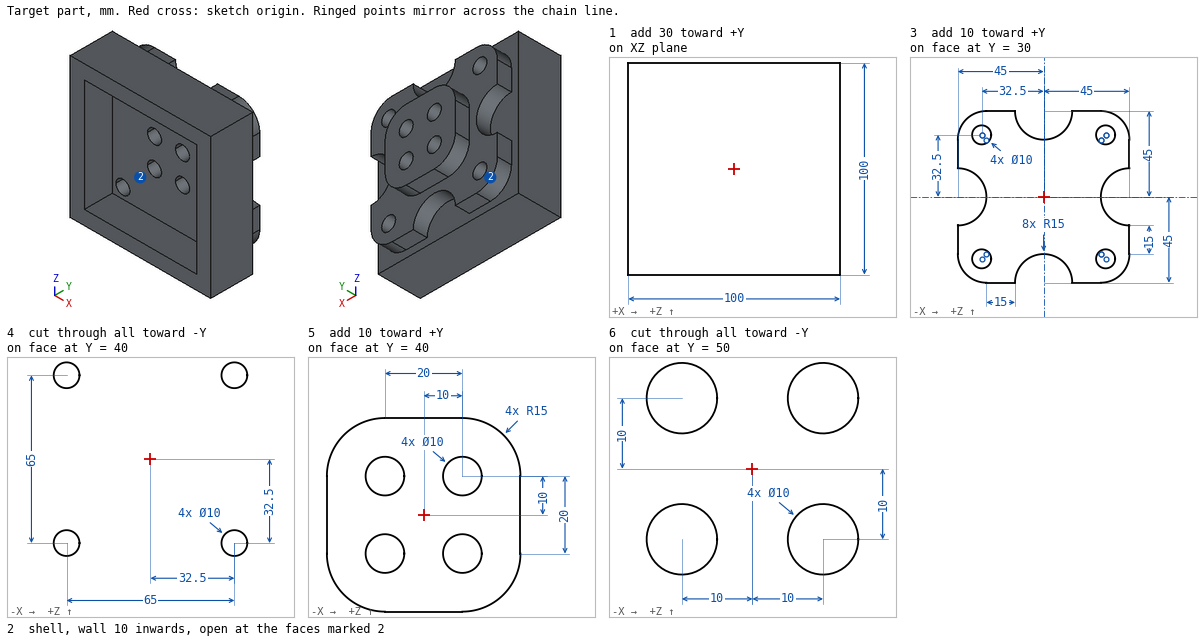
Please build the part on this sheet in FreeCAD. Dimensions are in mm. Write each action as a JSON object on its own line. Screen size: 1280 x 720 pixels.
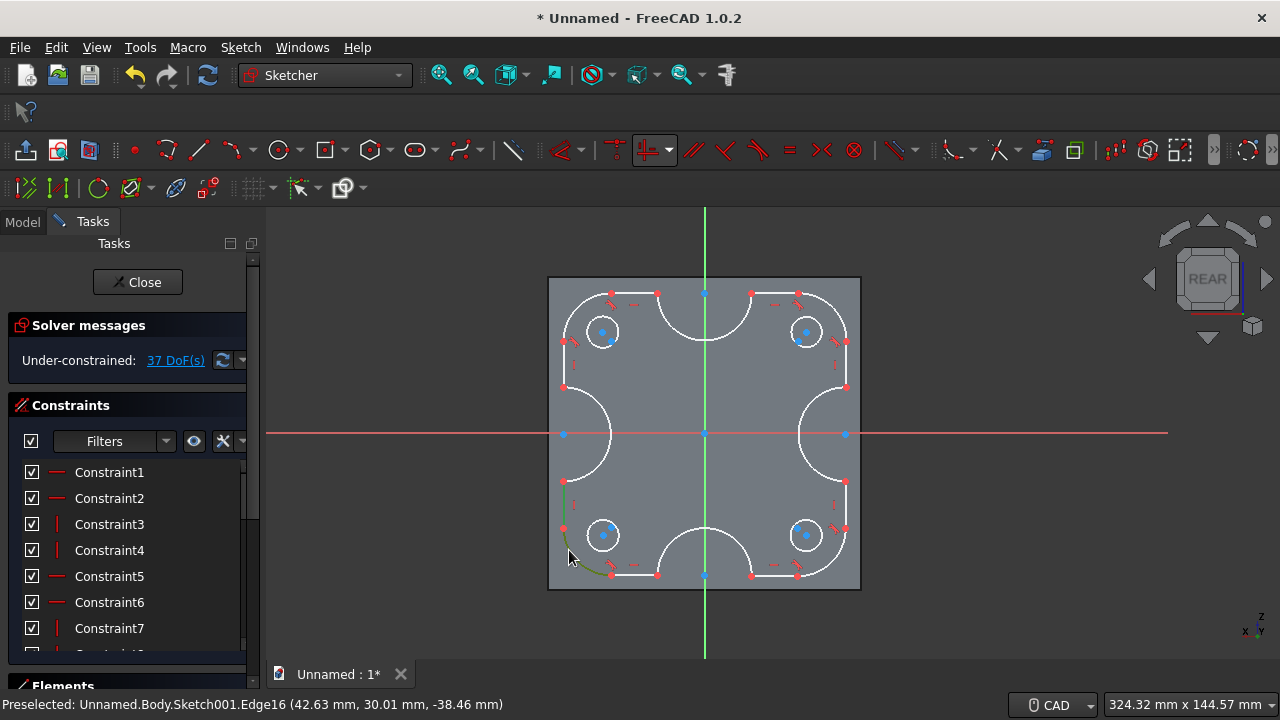
{"action": "left_click", "coordinate": [758, 150]}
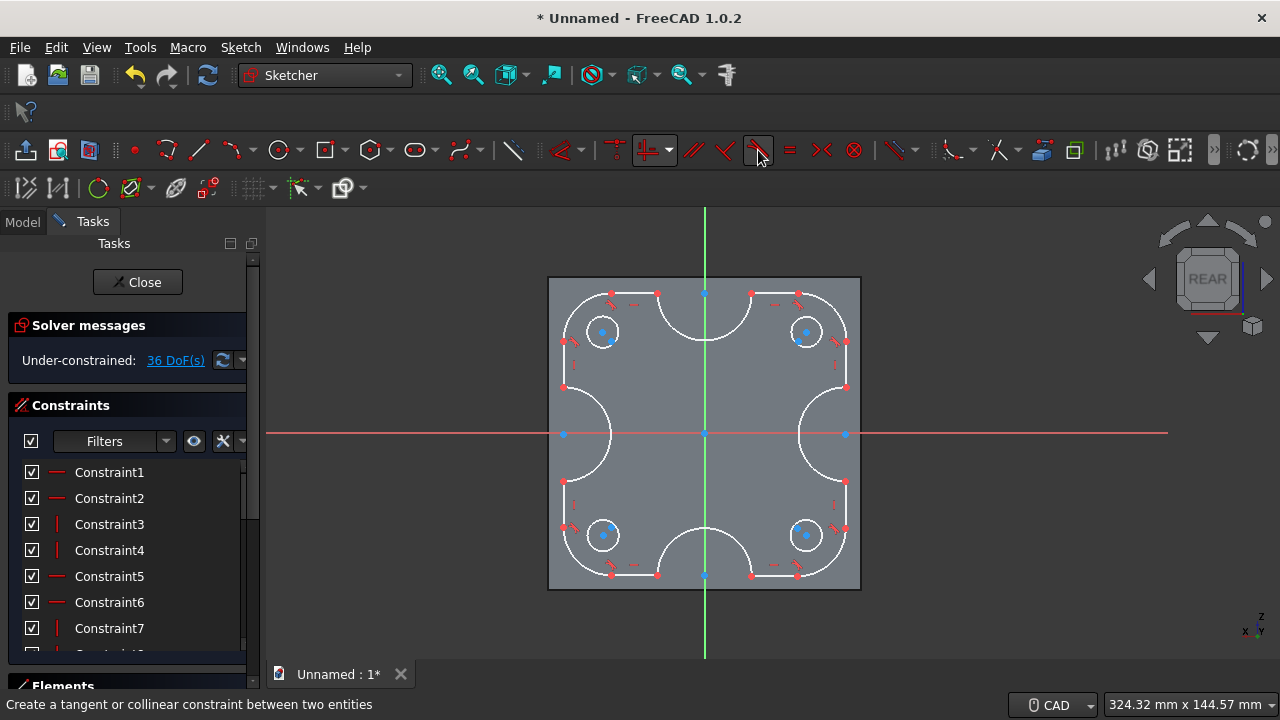
{"action": "left_click", "coordinate": [733, 538]}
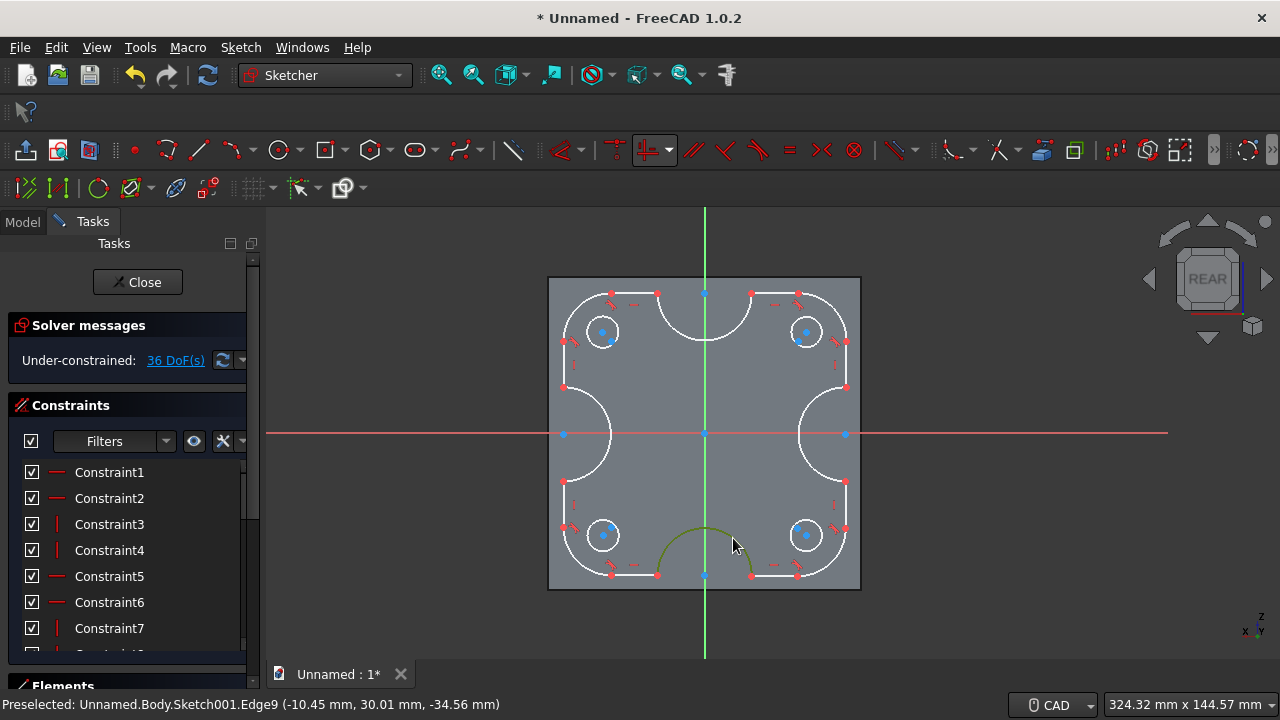
{"action": "left_click", "coordinate": [820, 571]}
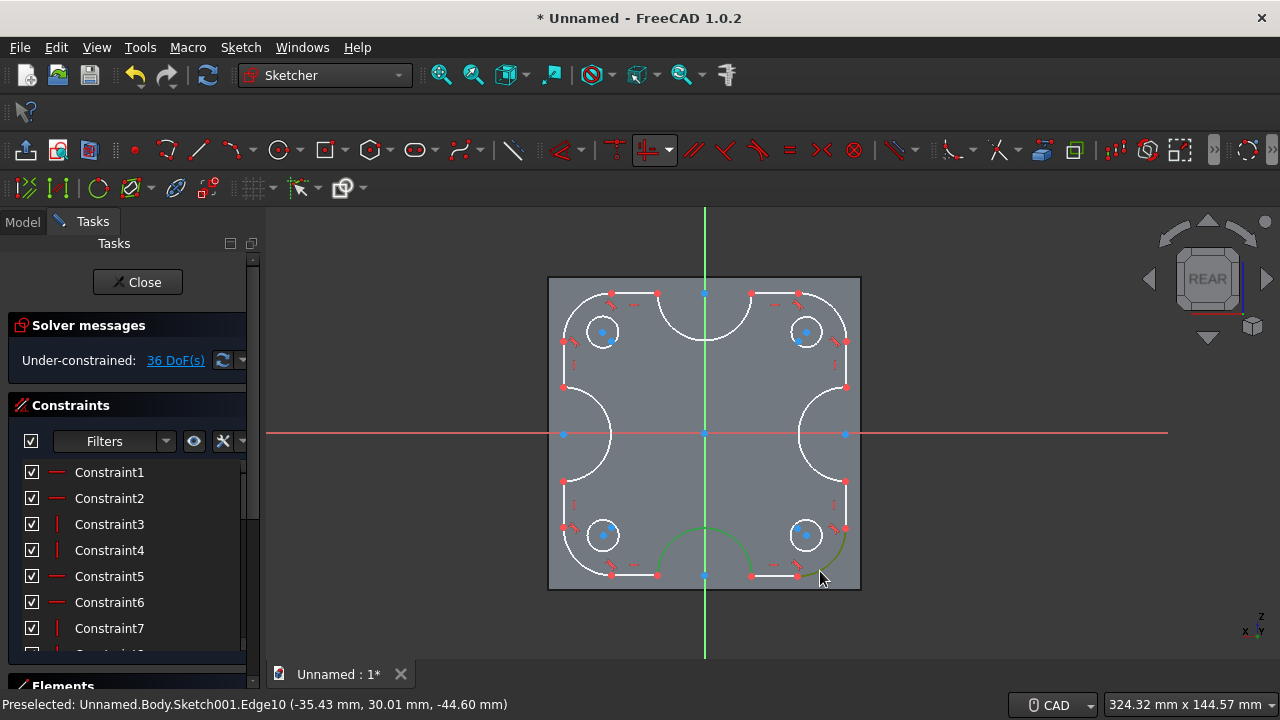
{"action": "left_click", "coordinate": [808, 406]}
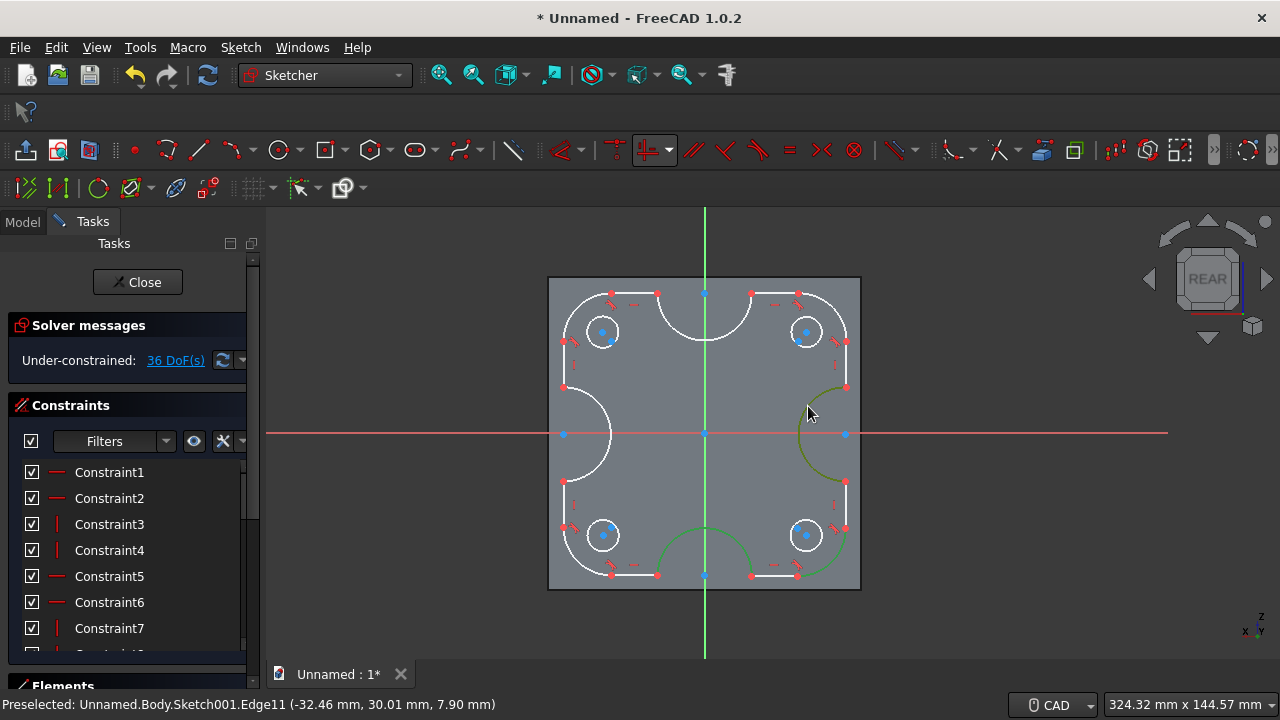
{"action": "left_click", "coordinate": [841, 319]}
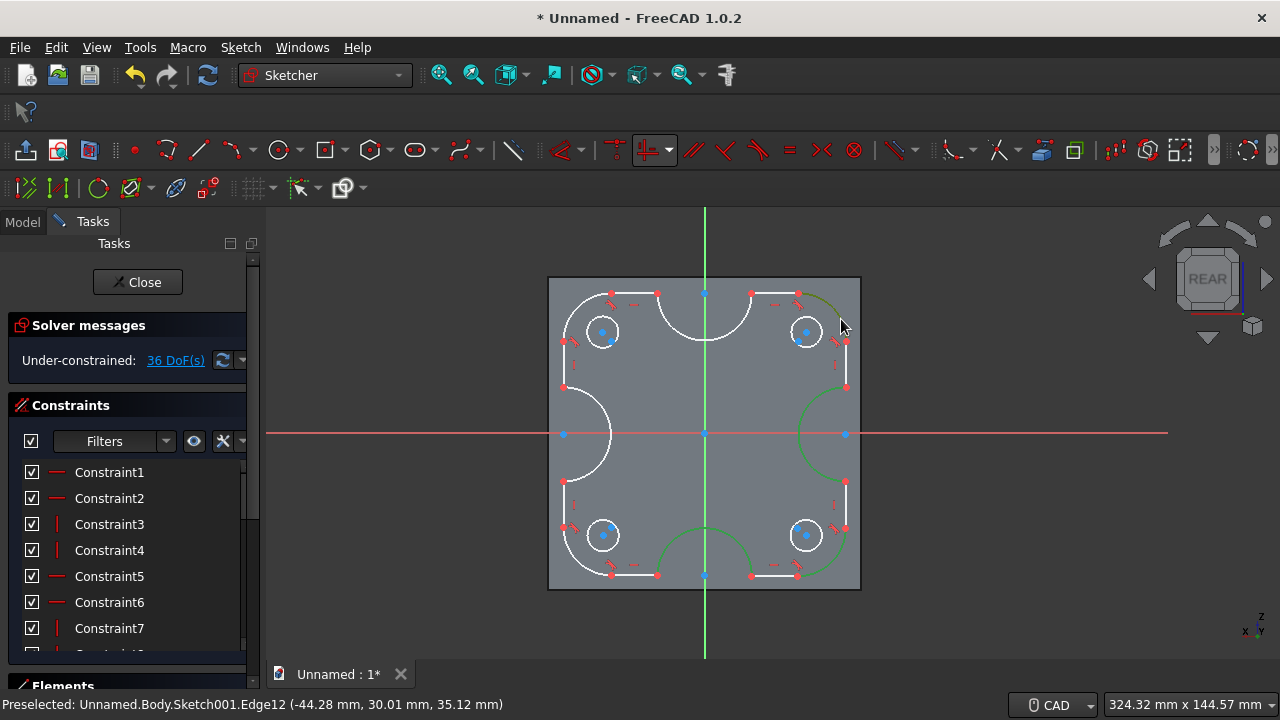
{"action": "left_click", "coordinate": [677, 331]}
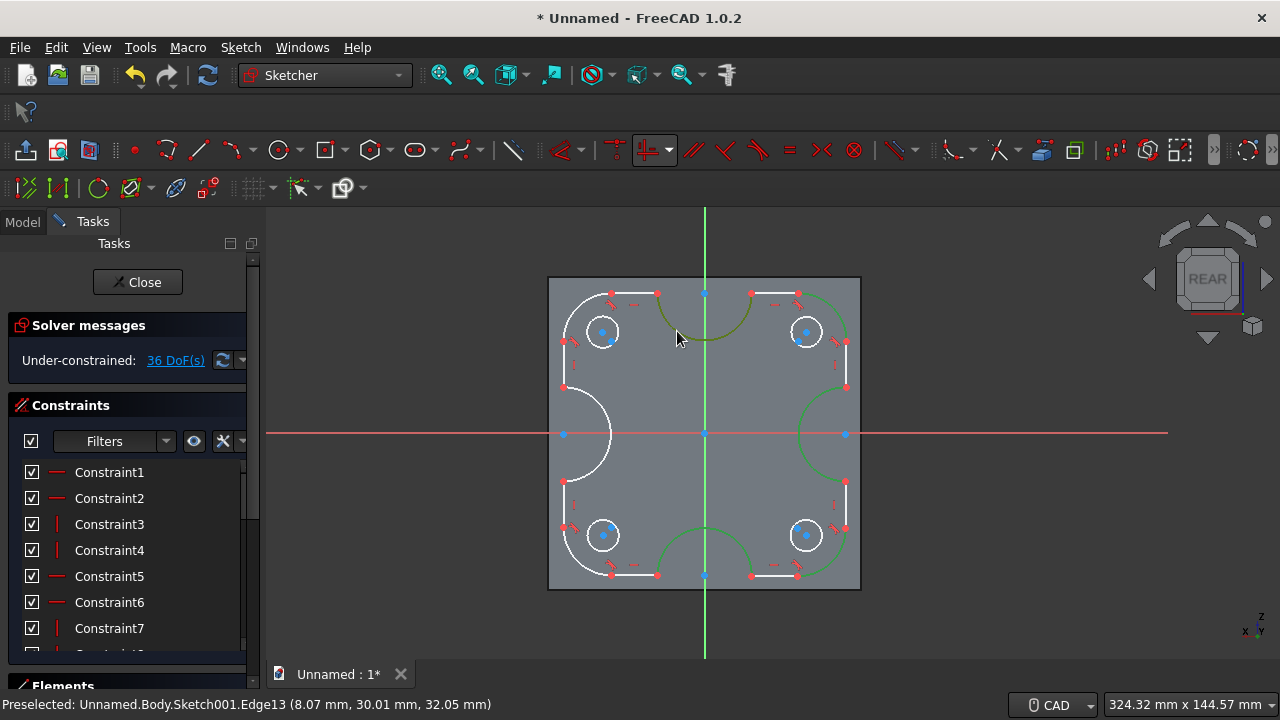
{"action": "left_click", "coordinate": [590, 299]}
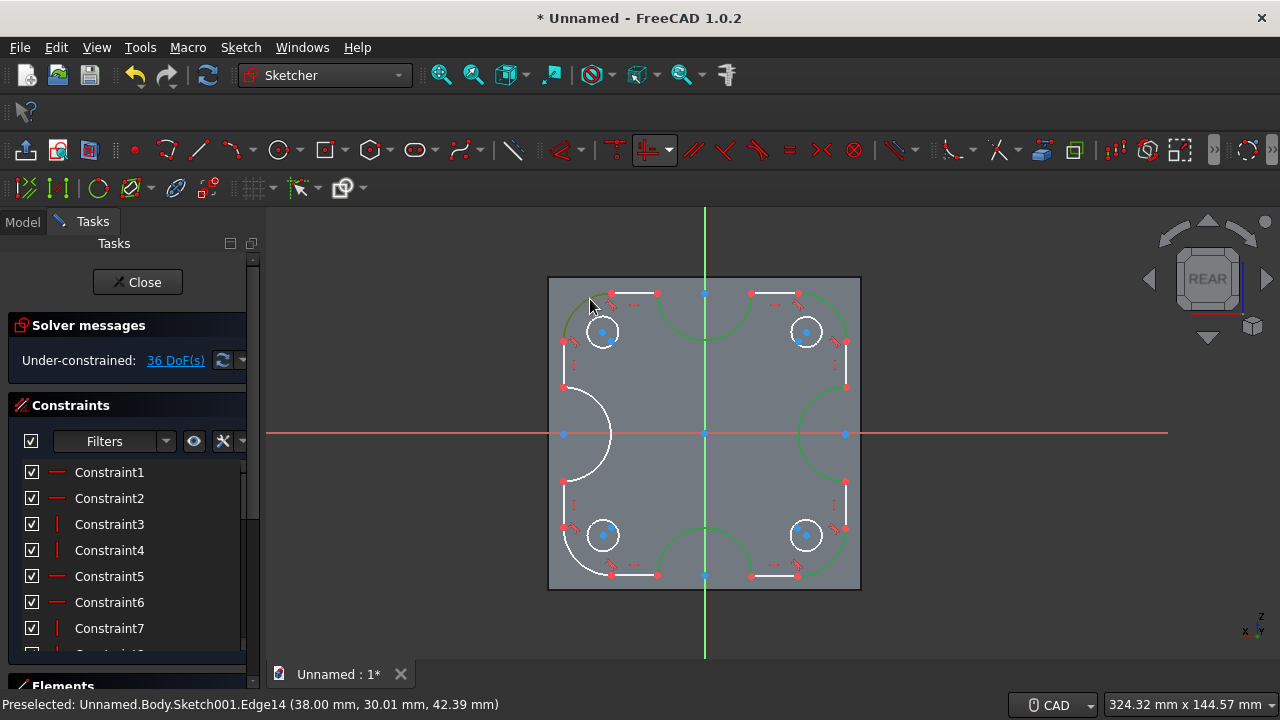
{"action": "left_click", "coordinate": [602, 462]}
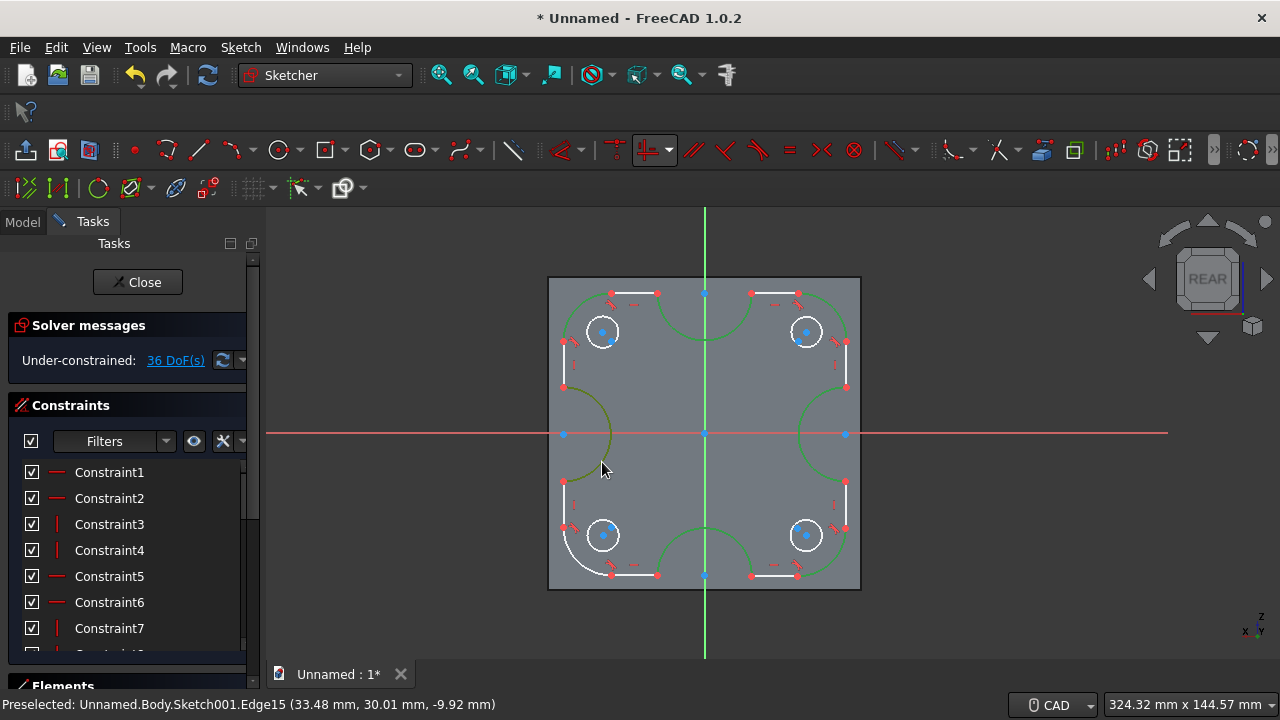
{"action": "left_click", "coordinate": [569, 549]}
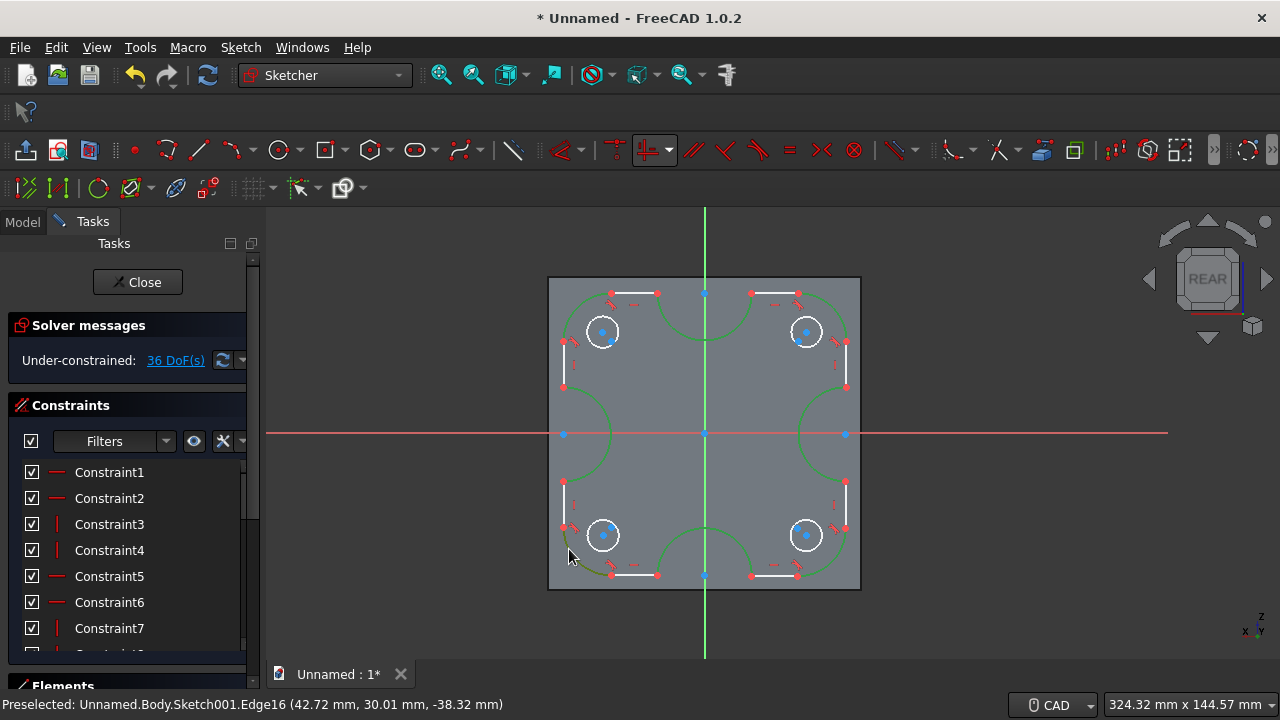
{"action": "left_click", "coordinate": [790, 150]}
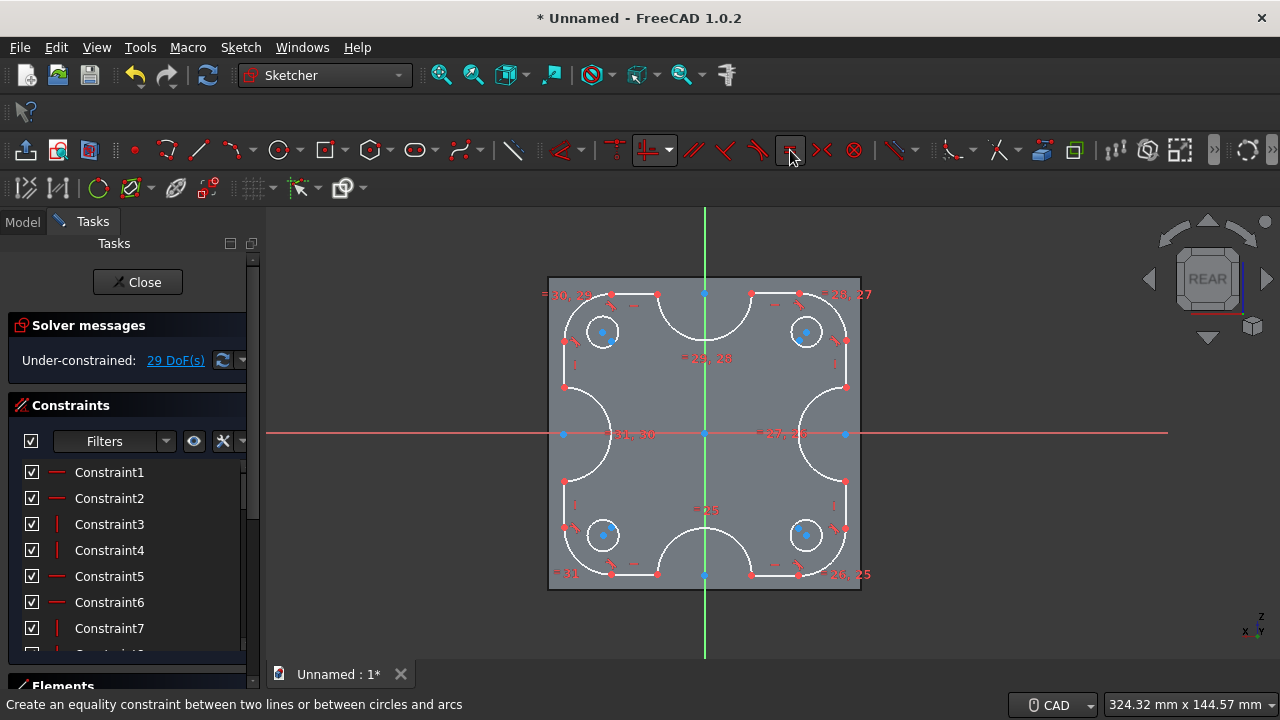
{"action": "left_click", "coordinate": [614, 321]}